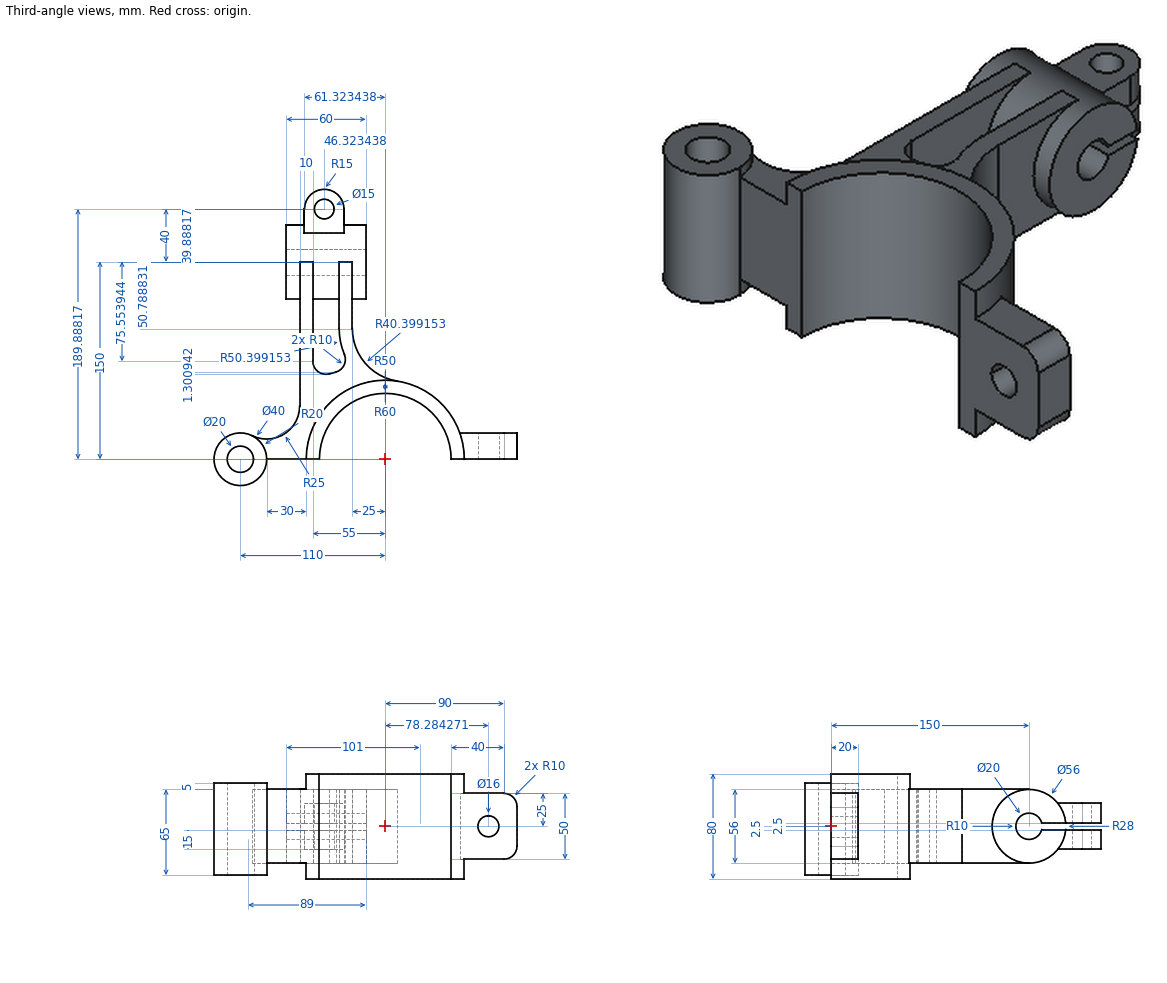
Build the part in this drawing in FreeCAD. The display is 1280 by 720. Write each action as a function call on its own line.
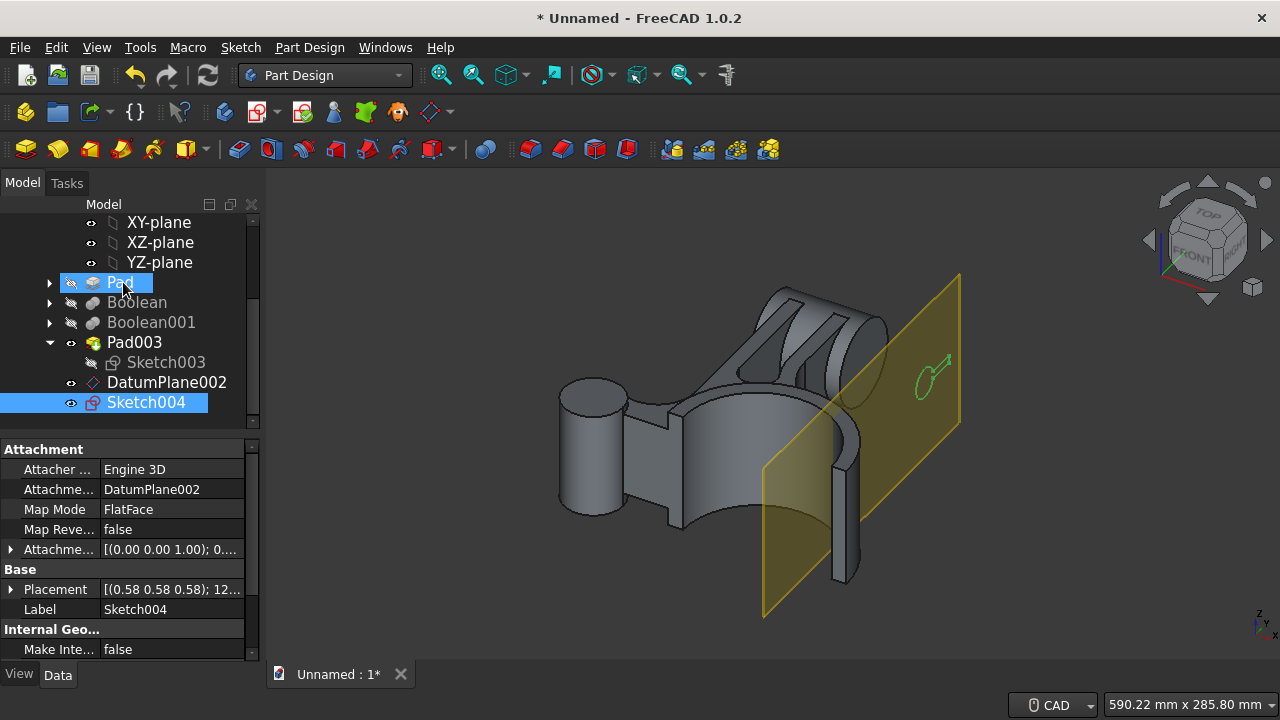
click(240, 150)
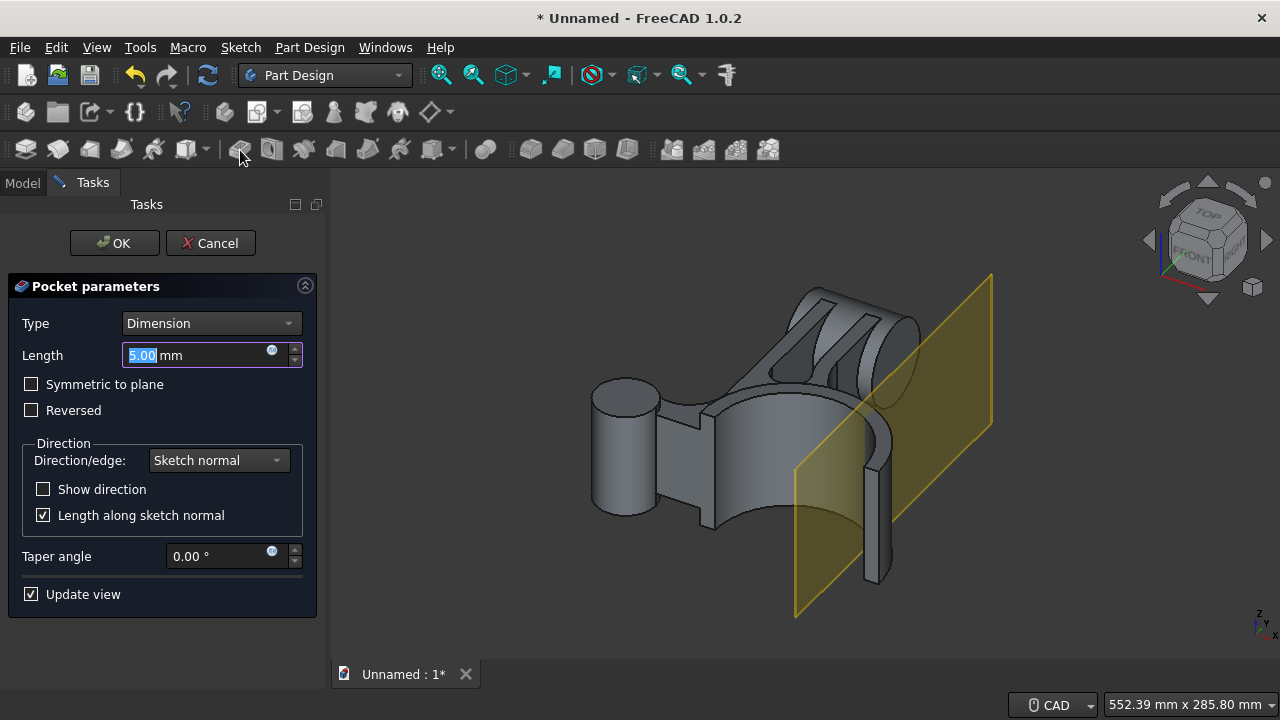
text(101)
key(Tab)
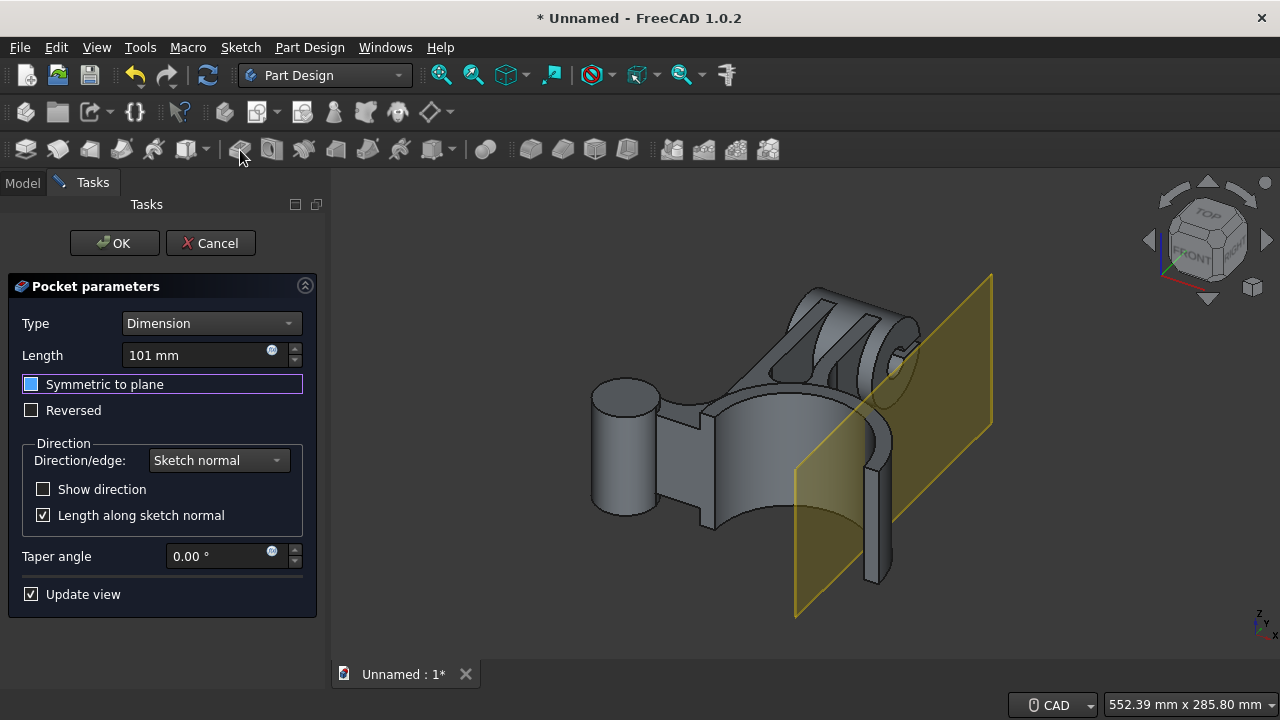
click(115, 243)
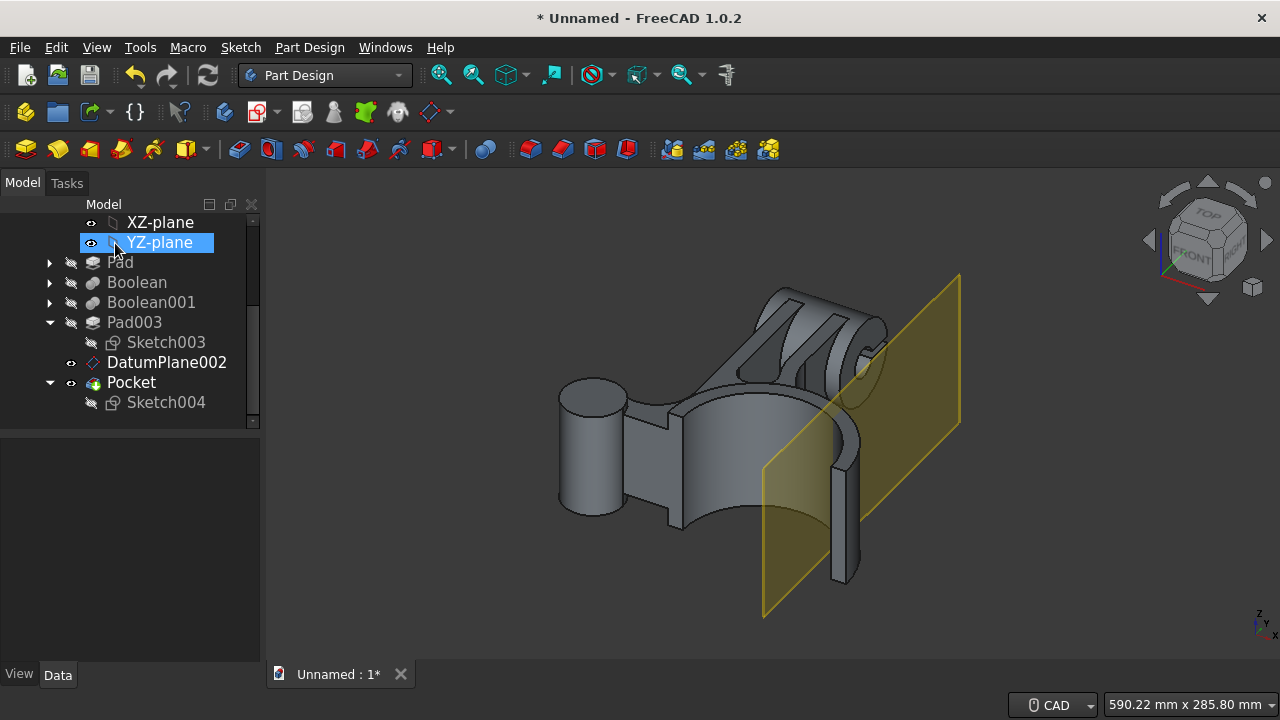
click(116, 363)
key(space)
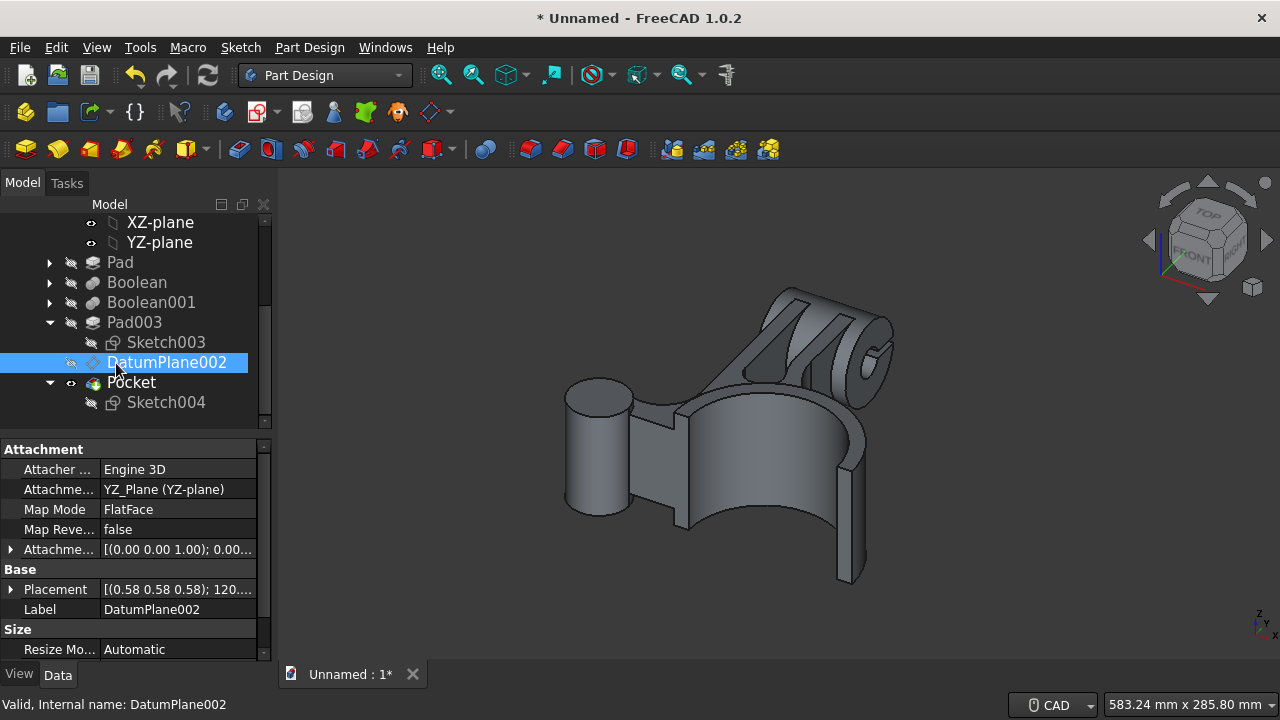
scroll(160, 318, down, 3)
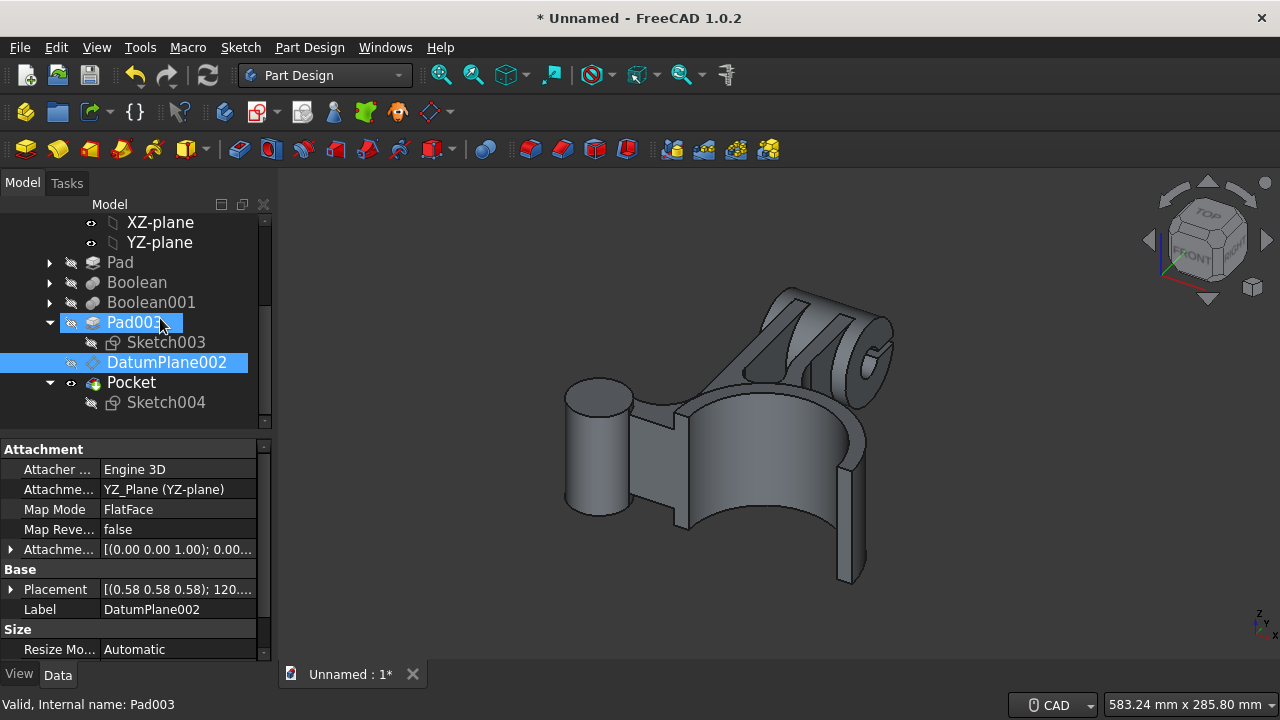
scroll(160, 318, up, 15)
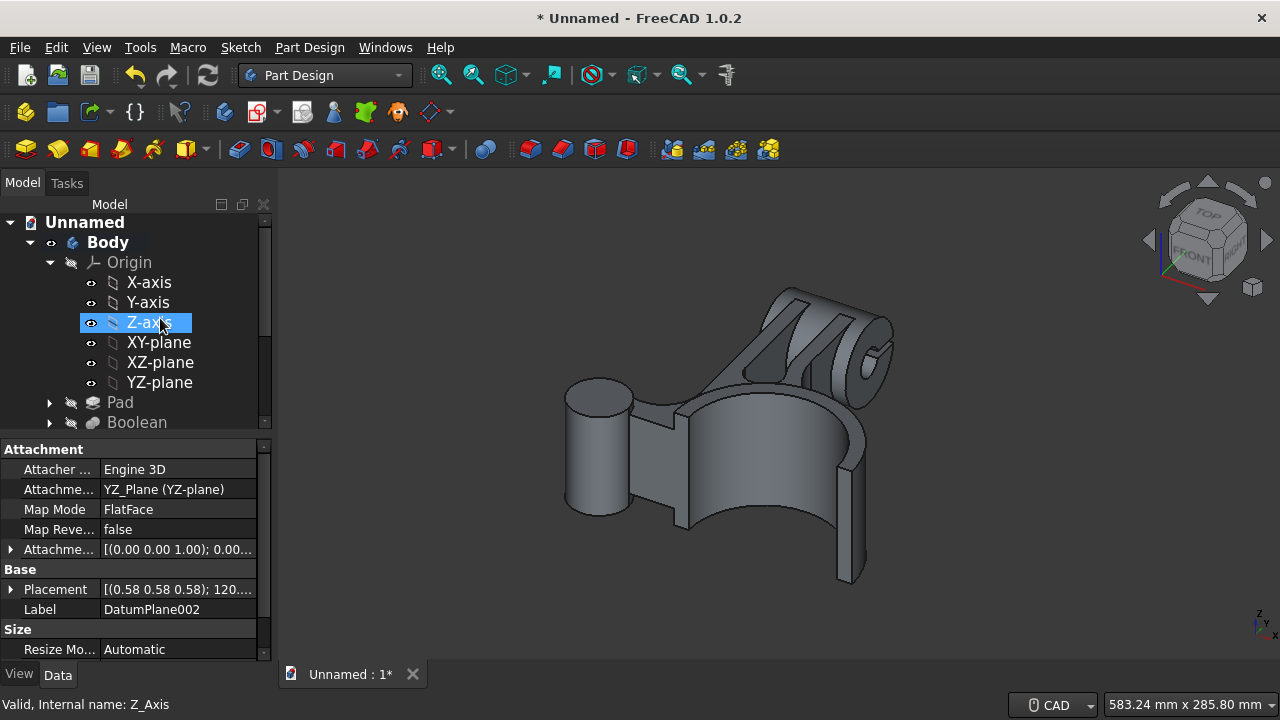
click(136, 343)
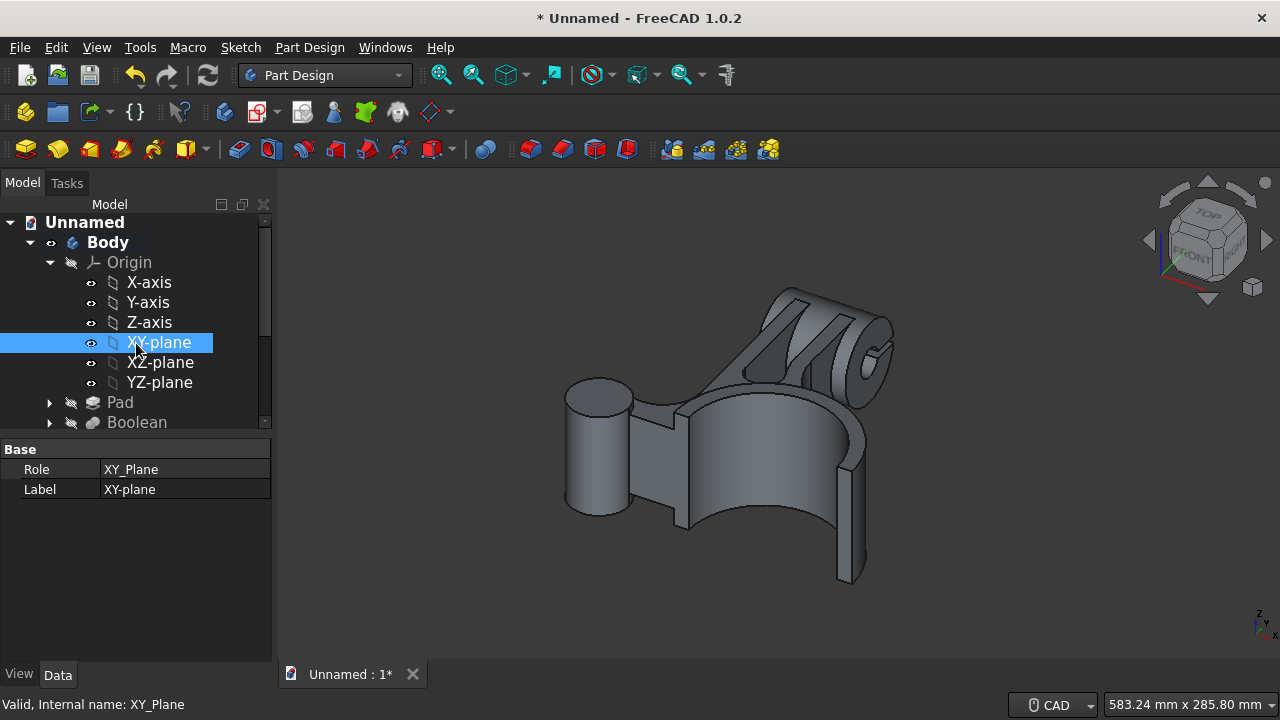
click(430, 112)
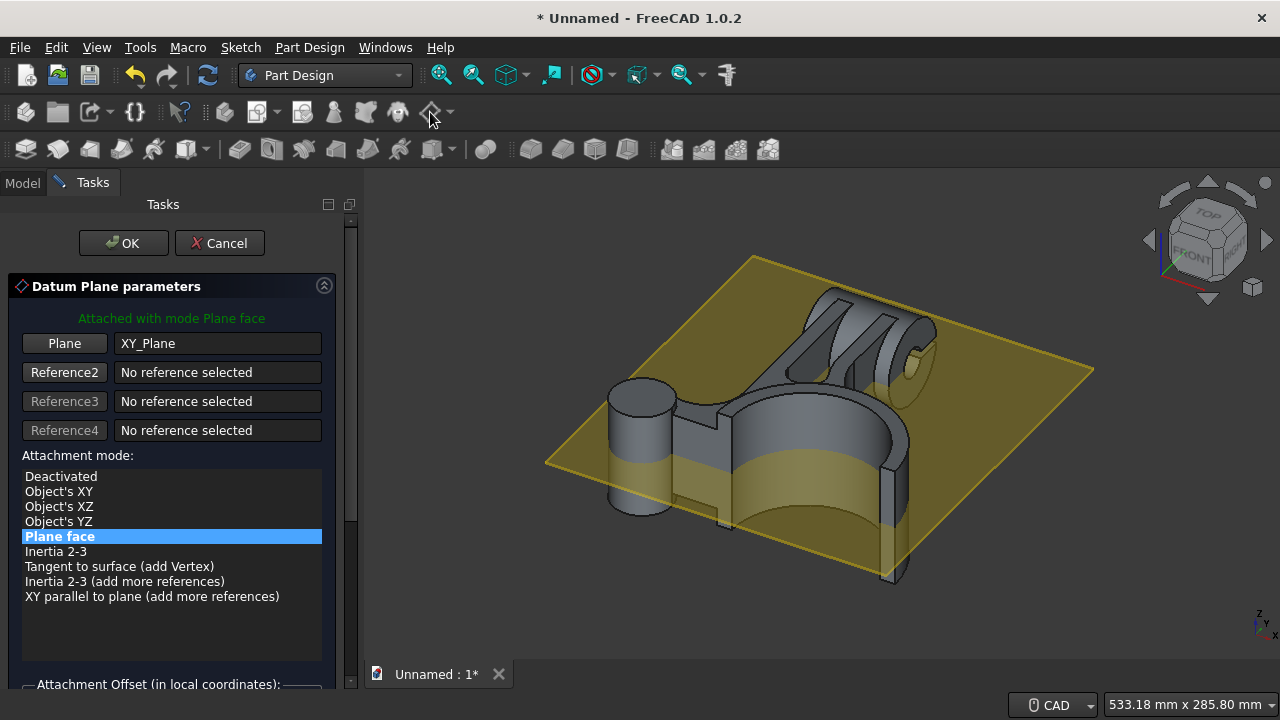
scroll(351, 451, down, 3)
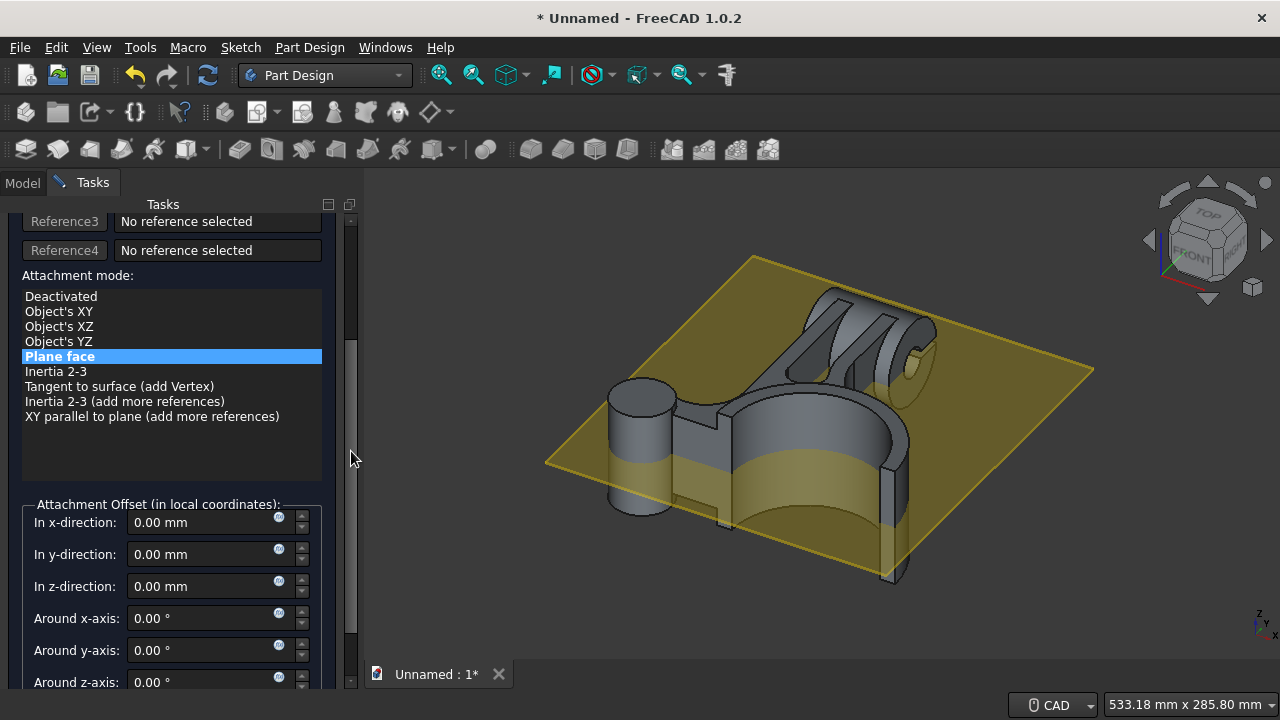
triple_click(210, 586)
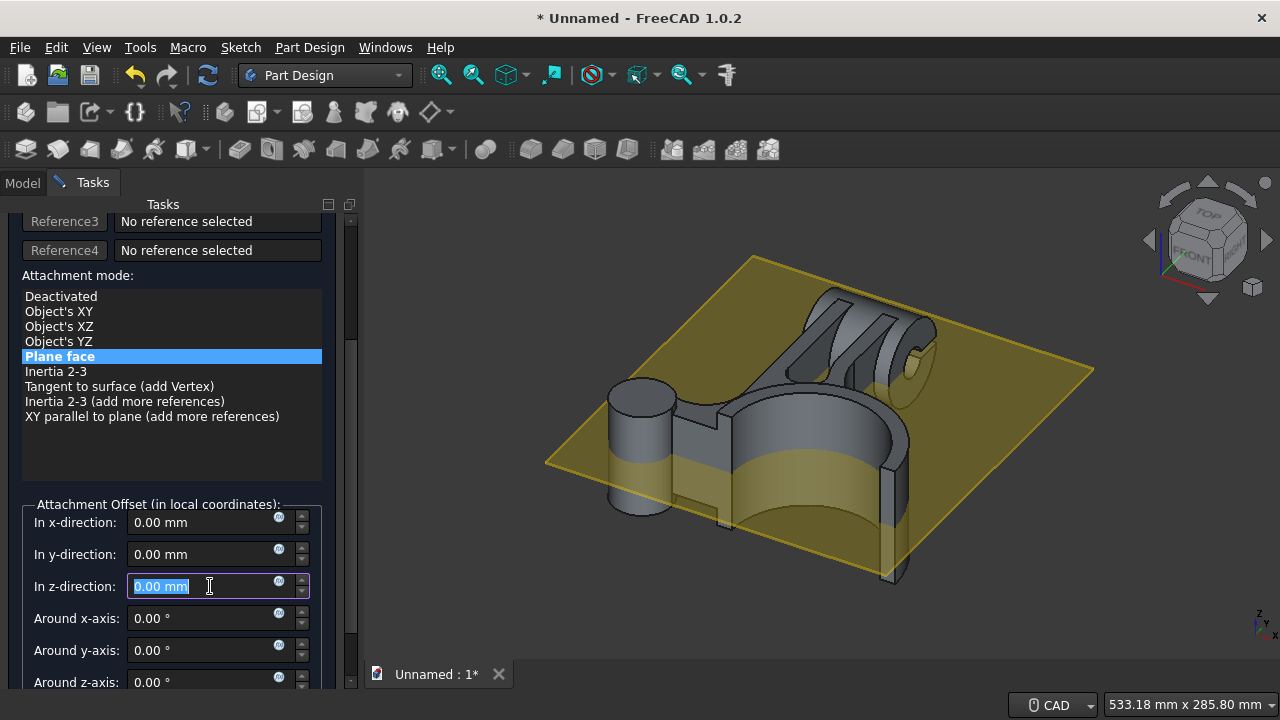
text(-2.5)
key(Tab)